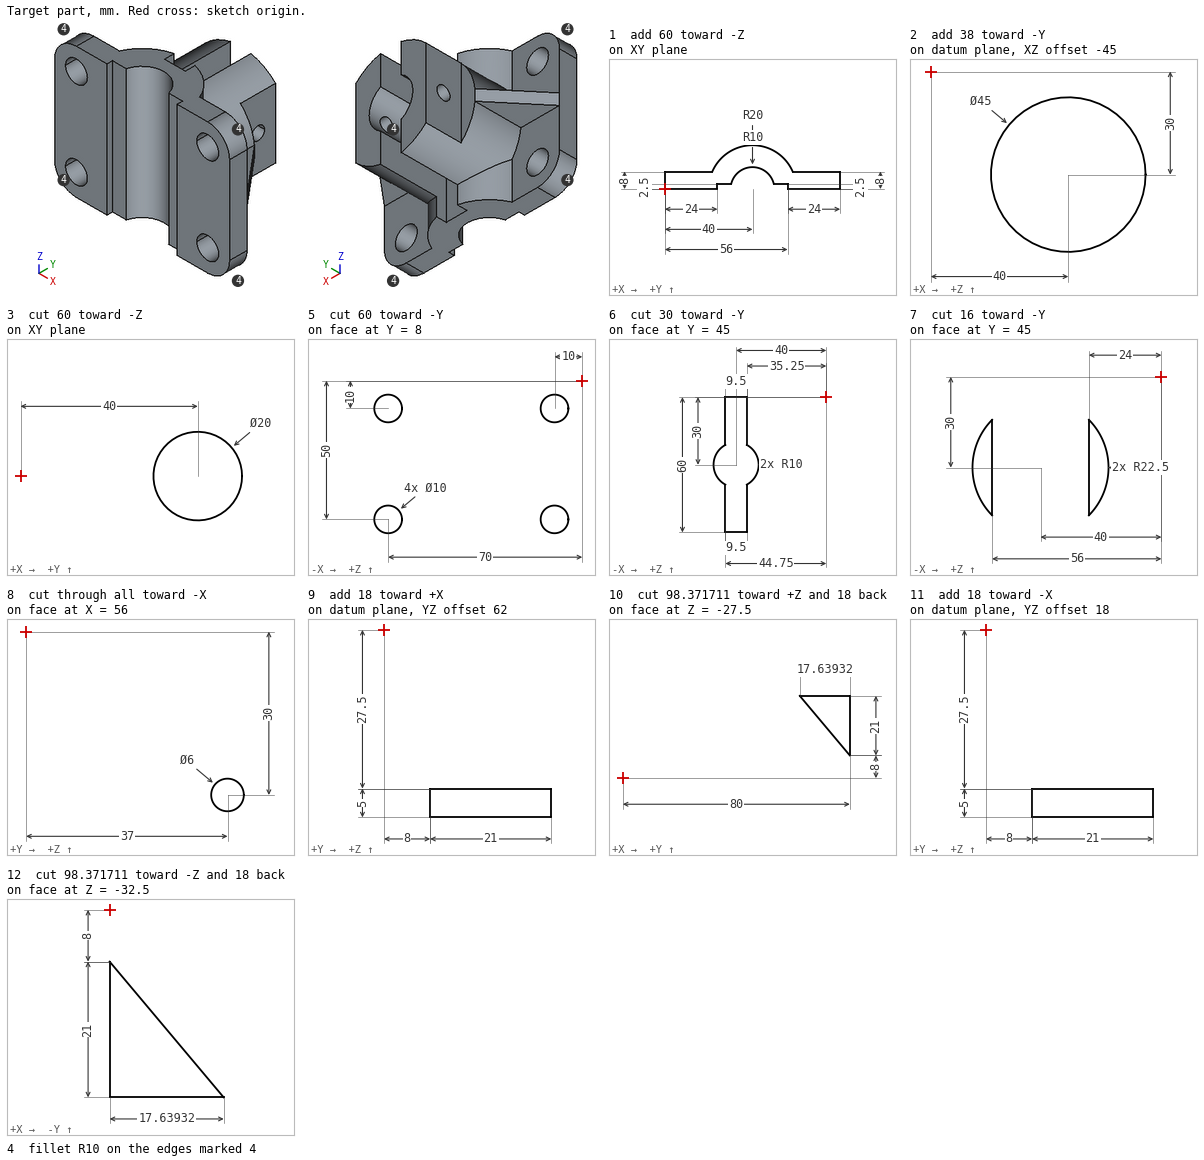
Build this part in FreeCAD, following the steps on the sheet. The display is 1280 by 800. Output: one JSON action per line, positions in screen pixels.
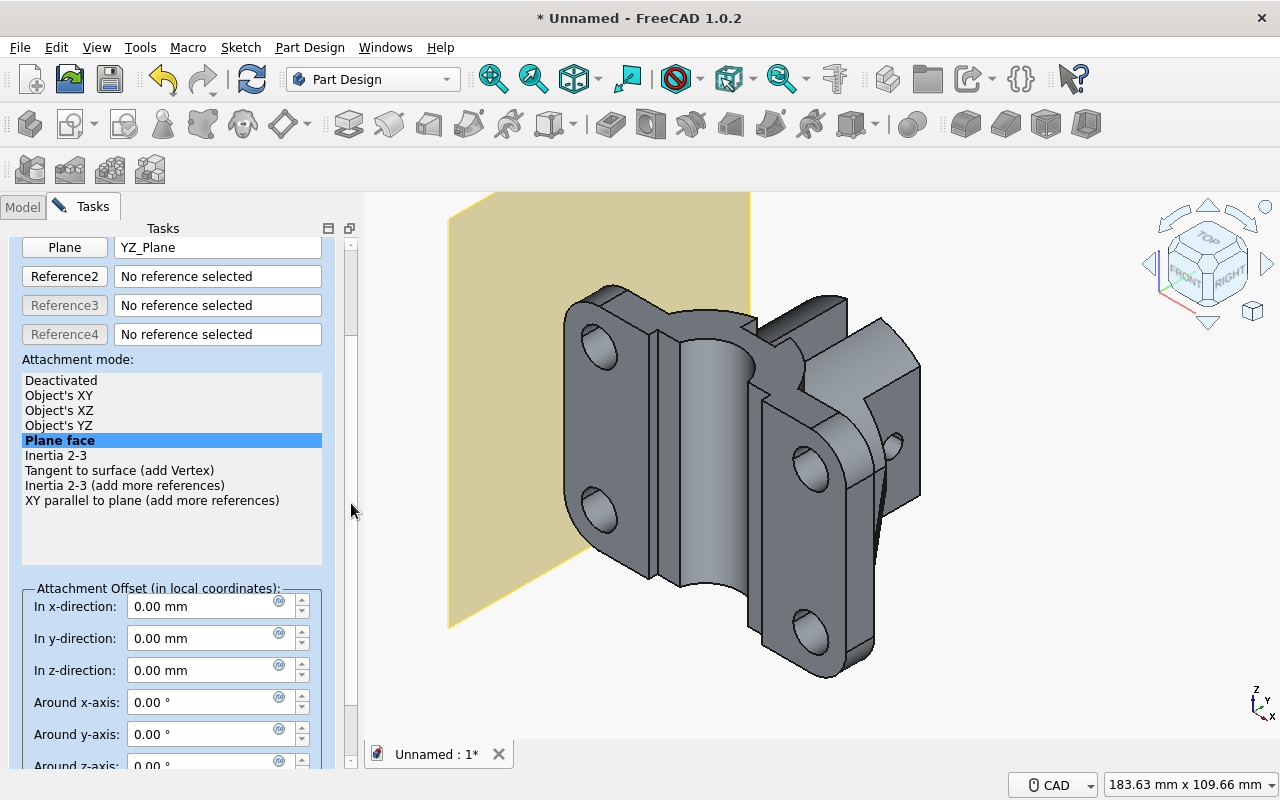
{"action": "triple_click", "coordinate": [210, 670]}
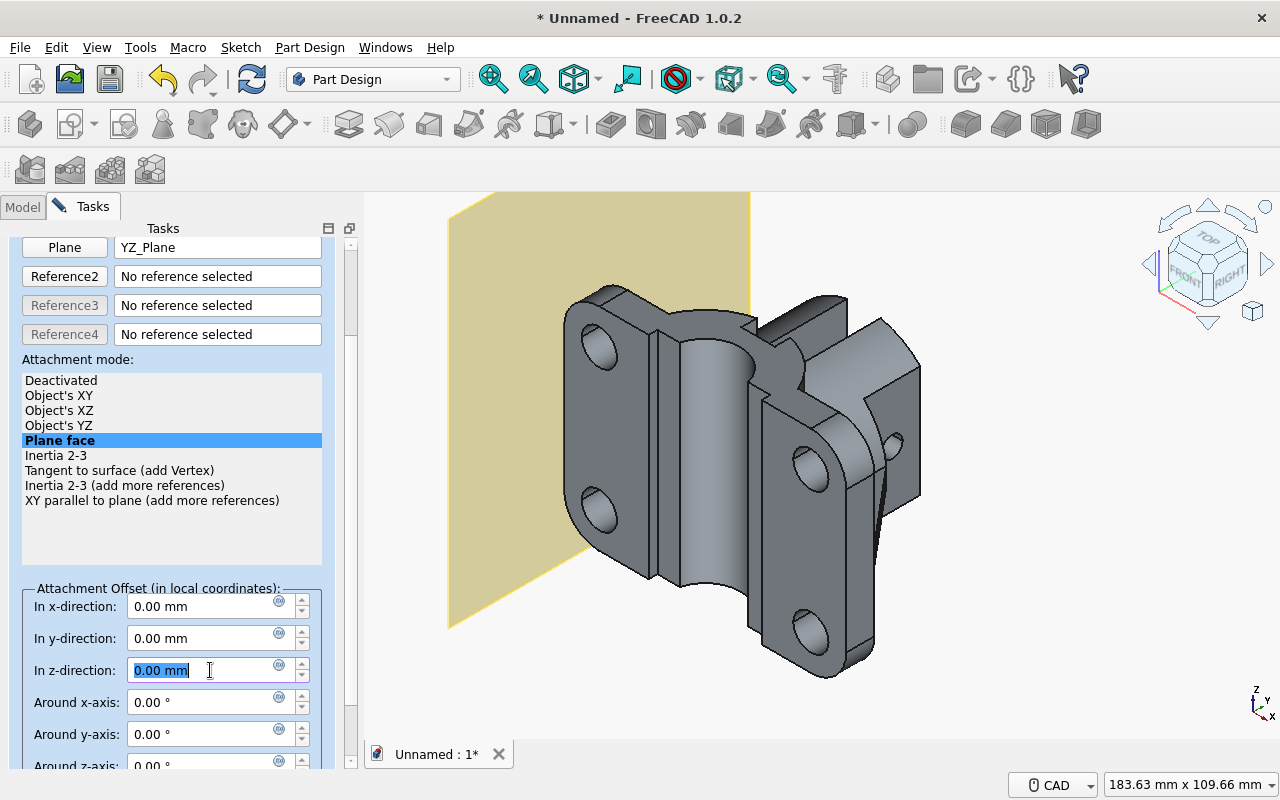
{"action": "type", "text": "18"}
{"action": "key", "text": "Tab"}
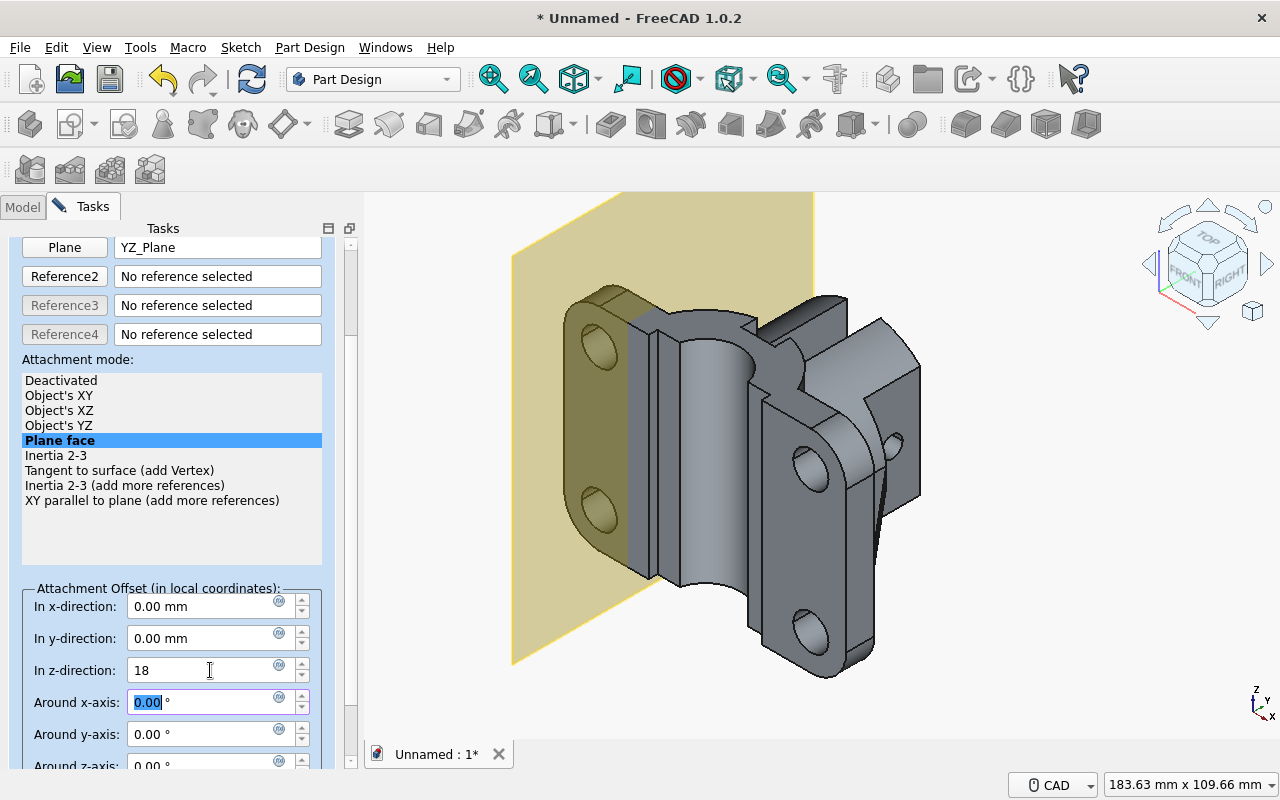
{"action": "scroll", "coordinate": [351, 503], "scroll_direction": "up", "scroll_amount": 3}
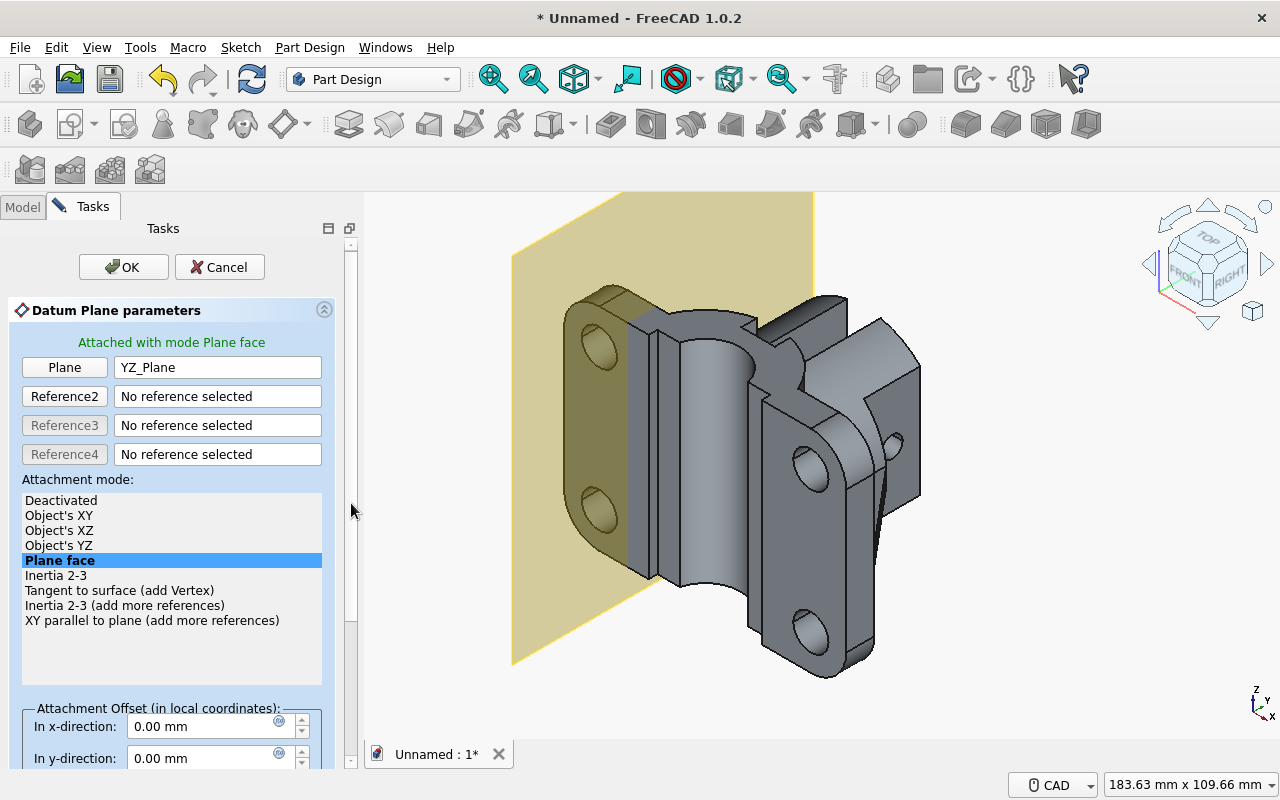
{"action": "left_click", "coordinate": [124, 267]}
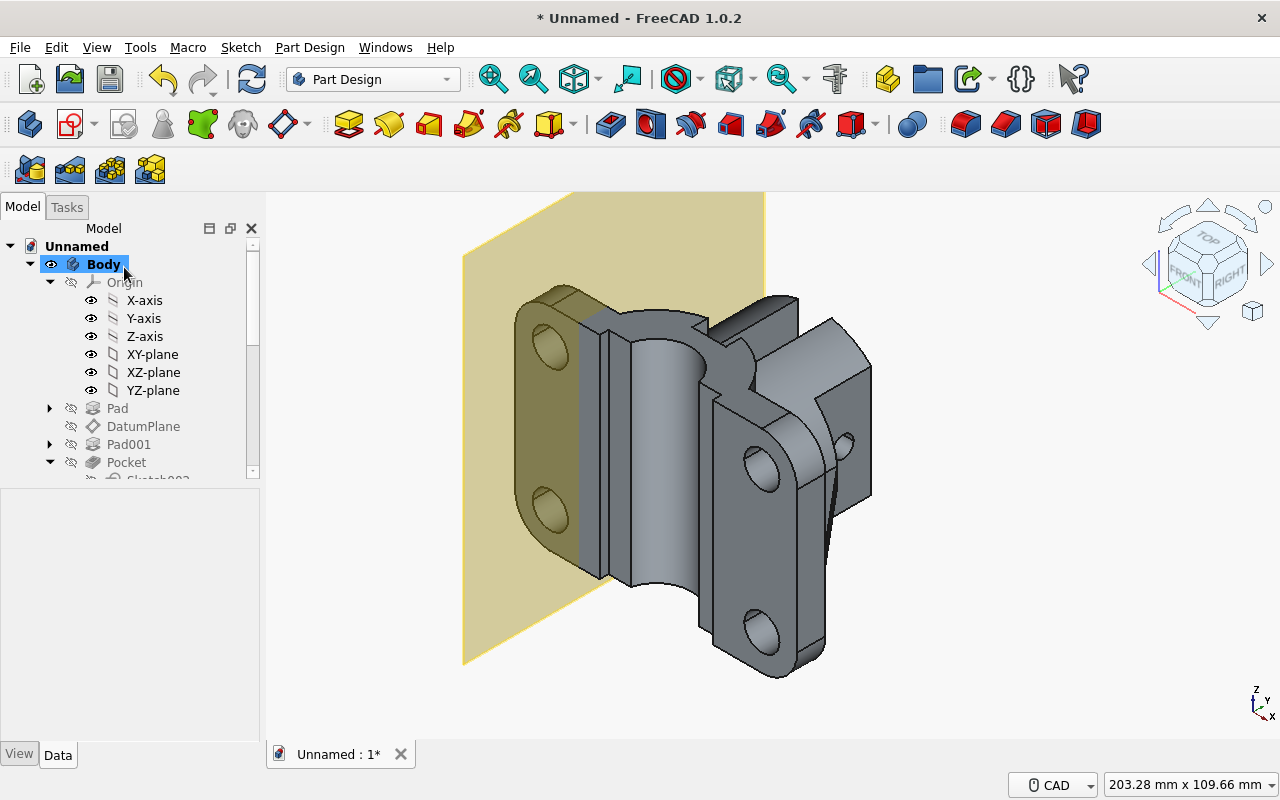
{"action": "scroll", "coordinate": [100, 350], "scroll_direction": "down", "scroll_amount": 3}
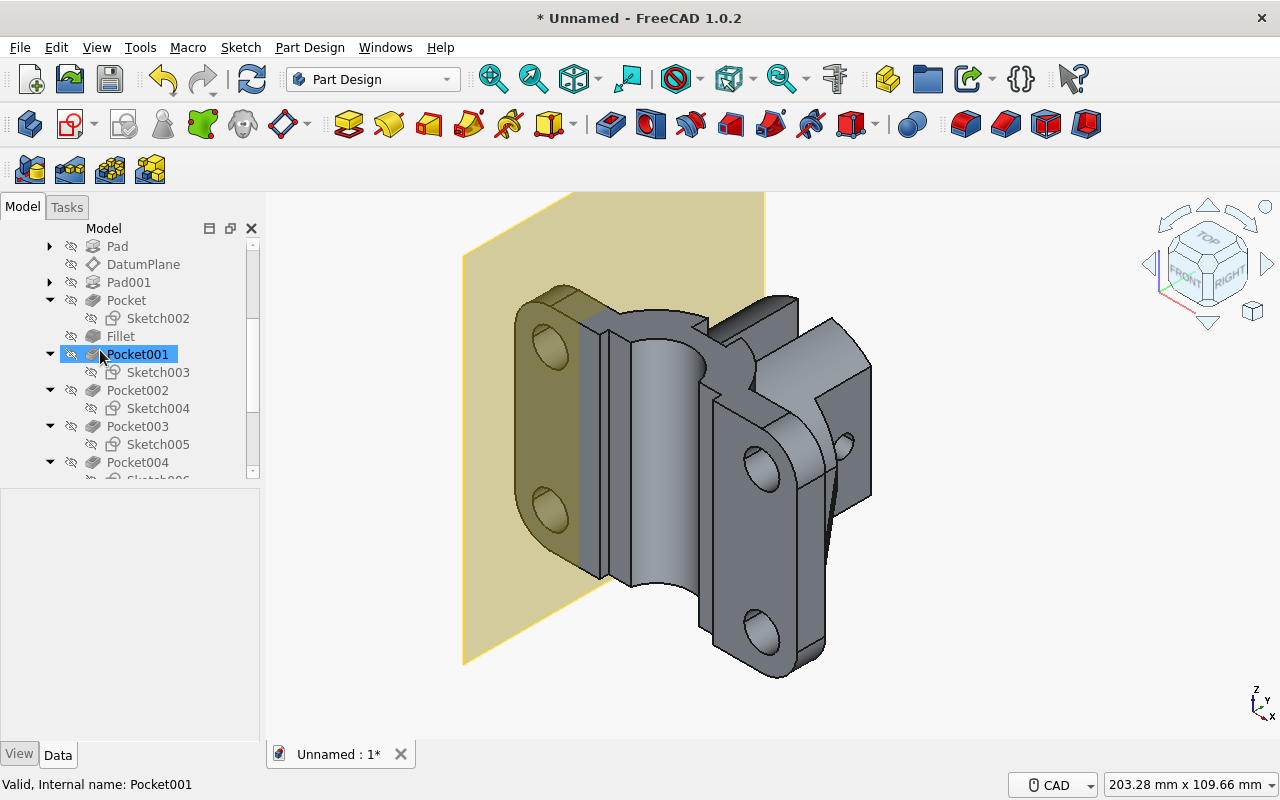
{"action": "scroll", "coordinate": [140, 350], "scroll_direction": "up", "scroll_amount": 15}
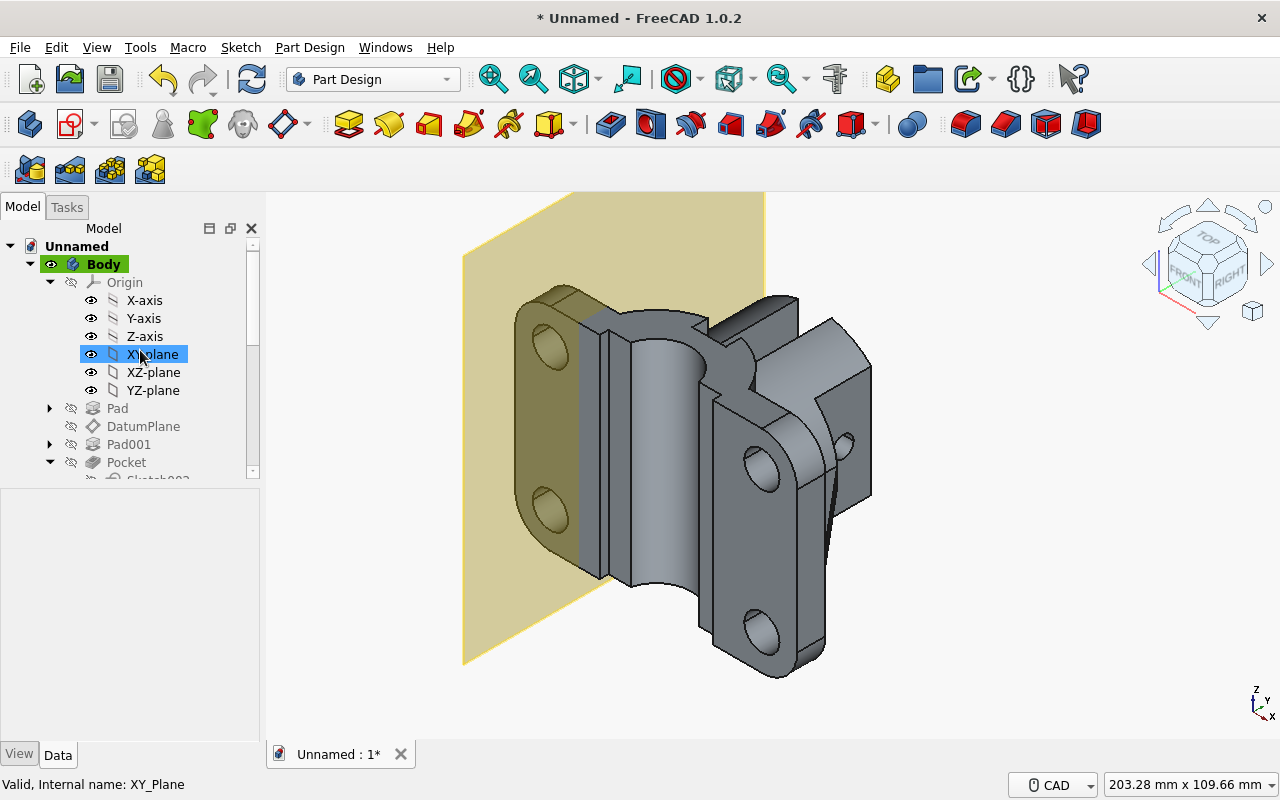
{"action": "scroll", "coordinate": [100, 350], "scroll_direction": "down", "scroll_amount": 6}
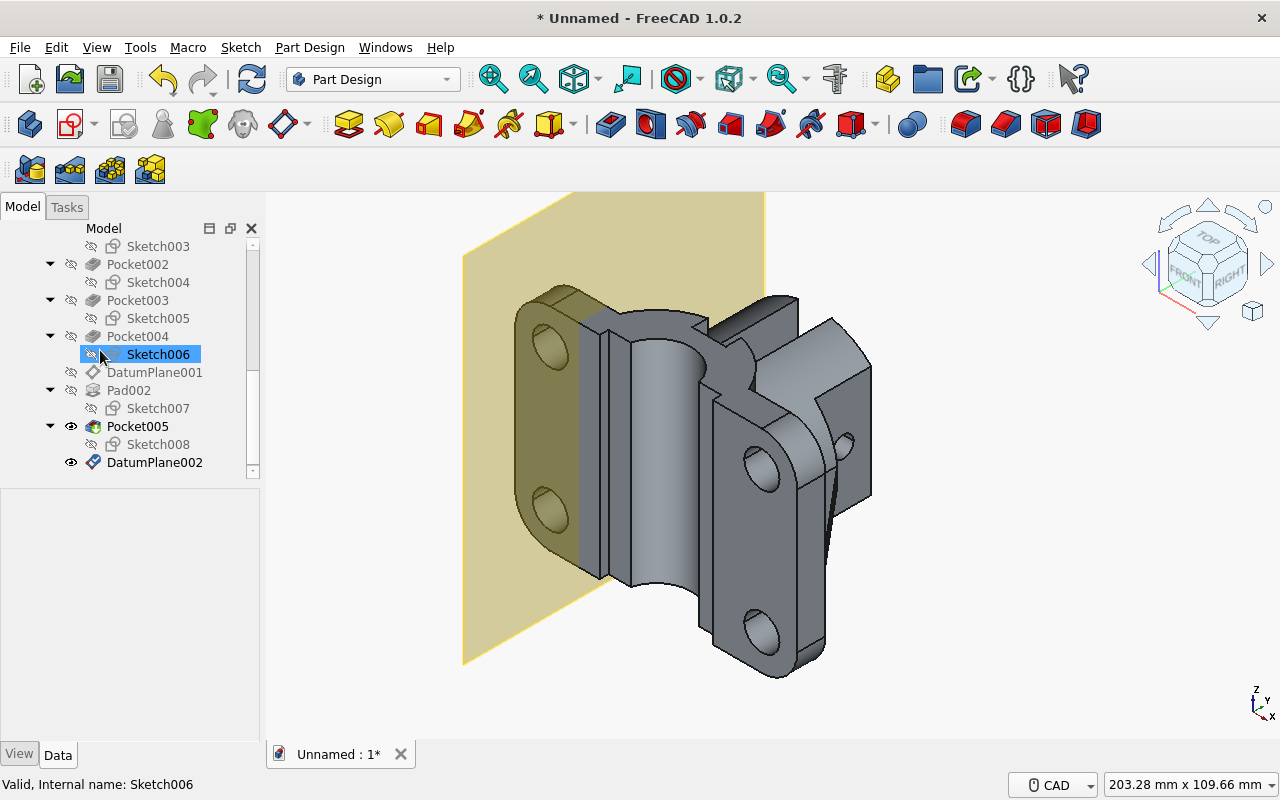
{"action": "left_click", "coordinate": [116, 462]}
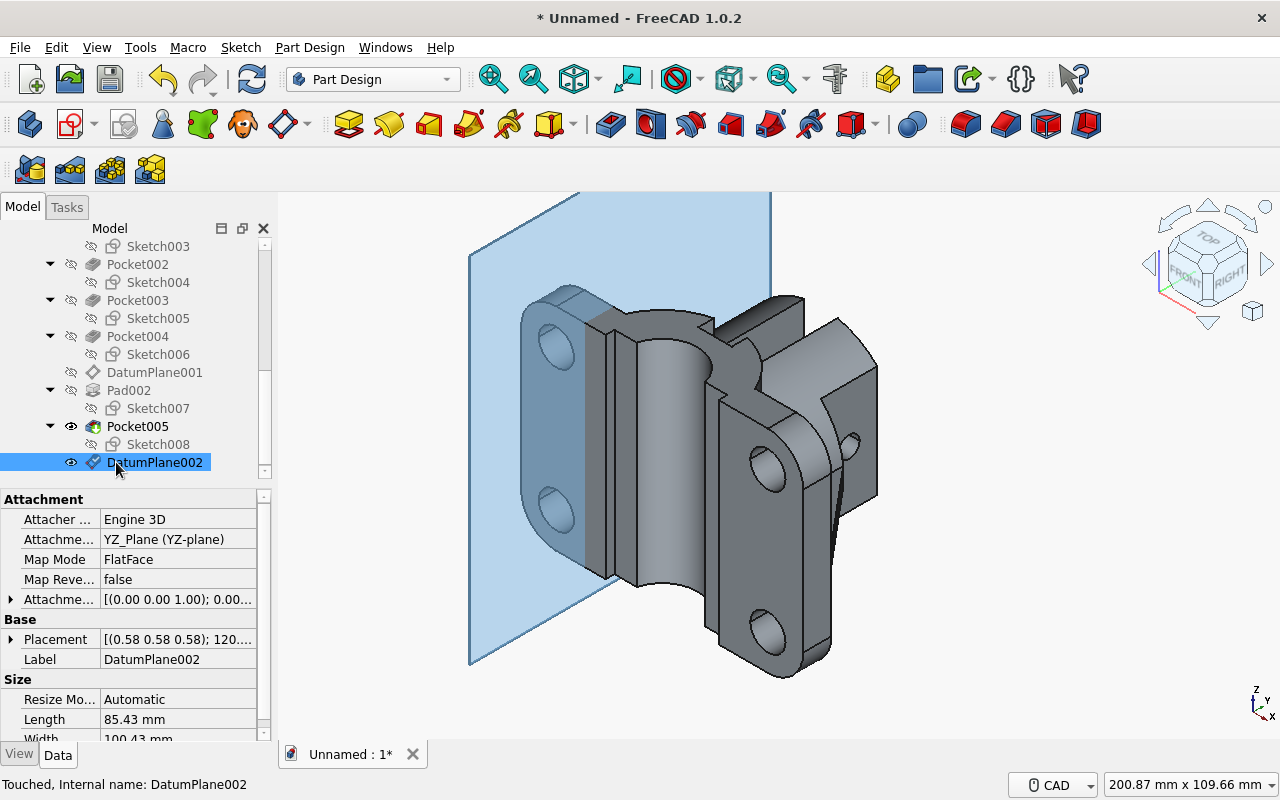
{"action": "left_click", "coordinate": [70, 124]}